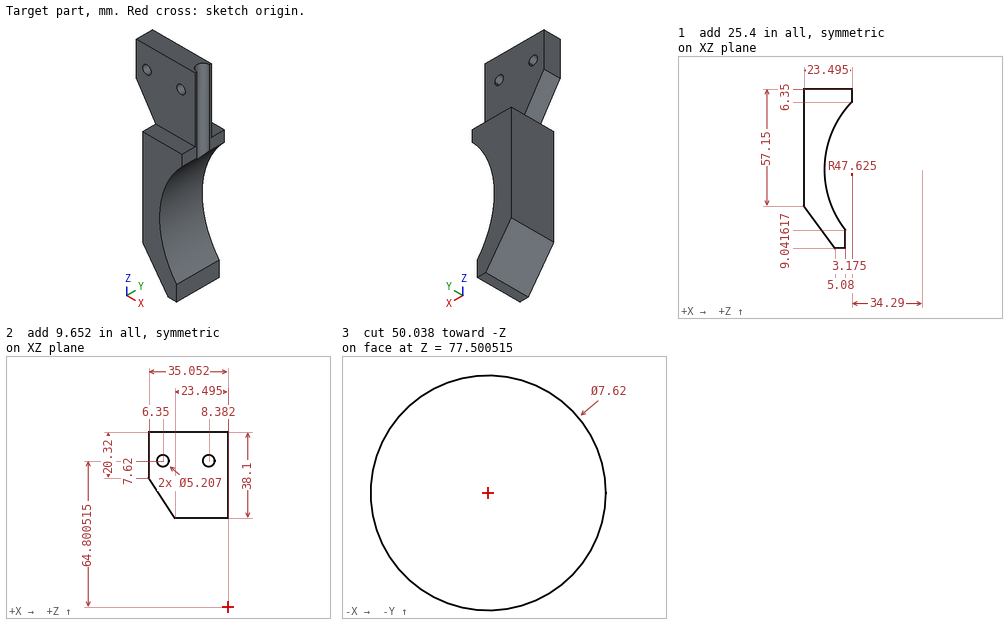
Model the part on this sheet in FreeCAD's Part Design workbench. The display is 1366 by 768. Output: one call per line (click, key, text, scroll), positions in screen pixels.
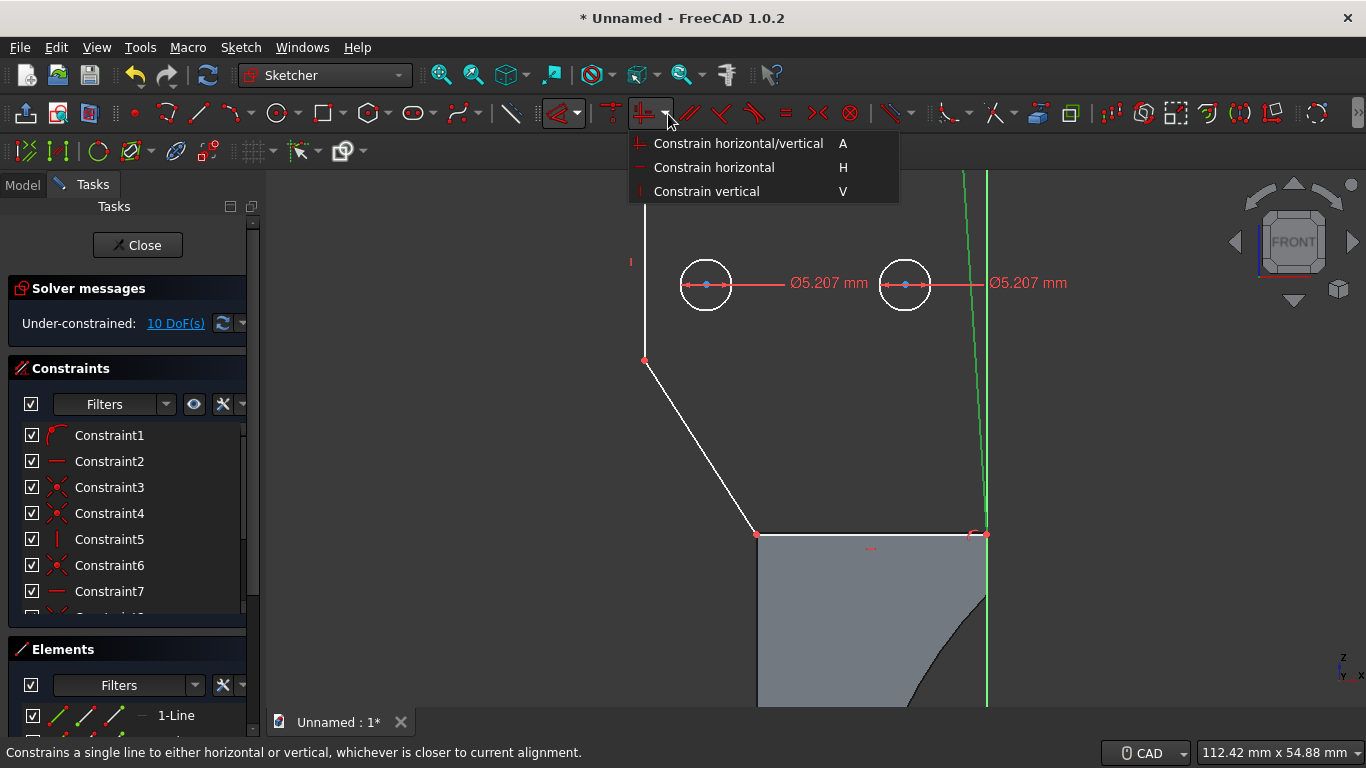
click(764, 191)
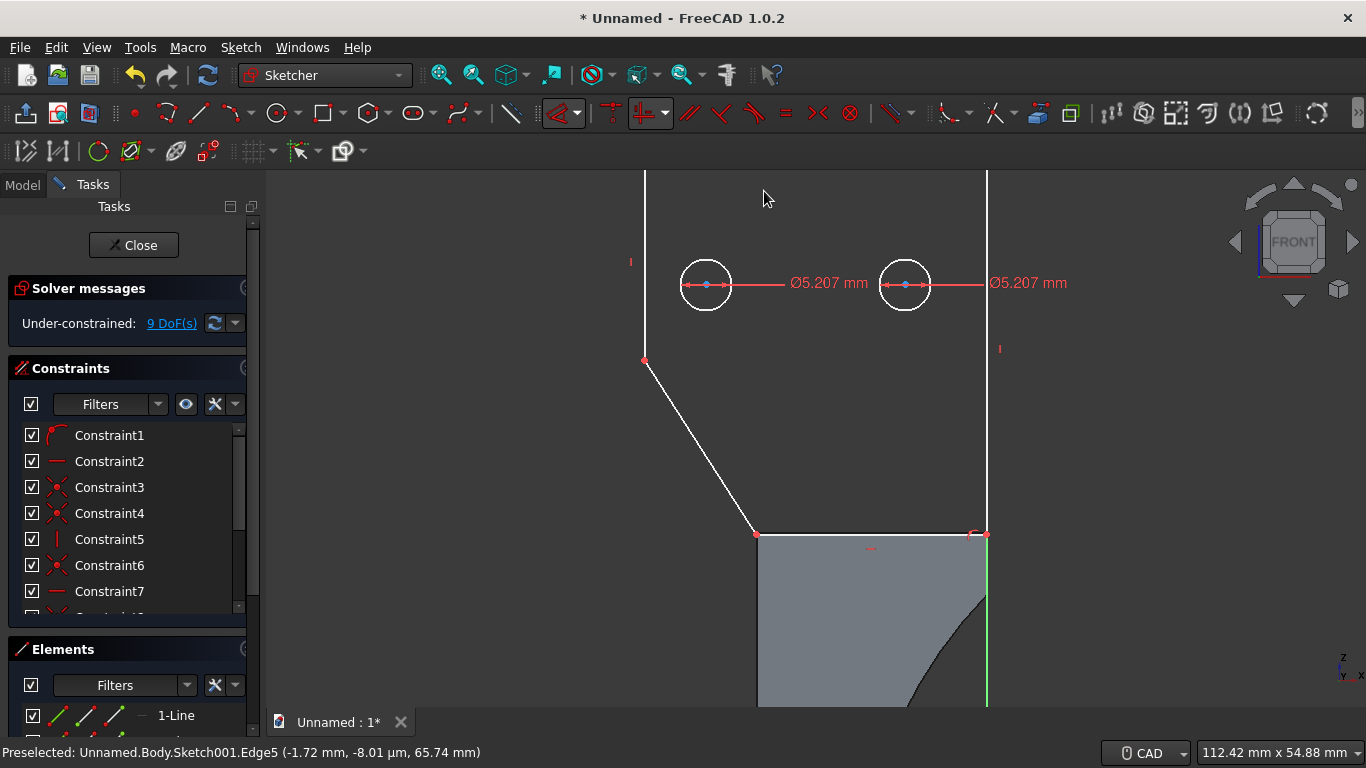
click(706, 285)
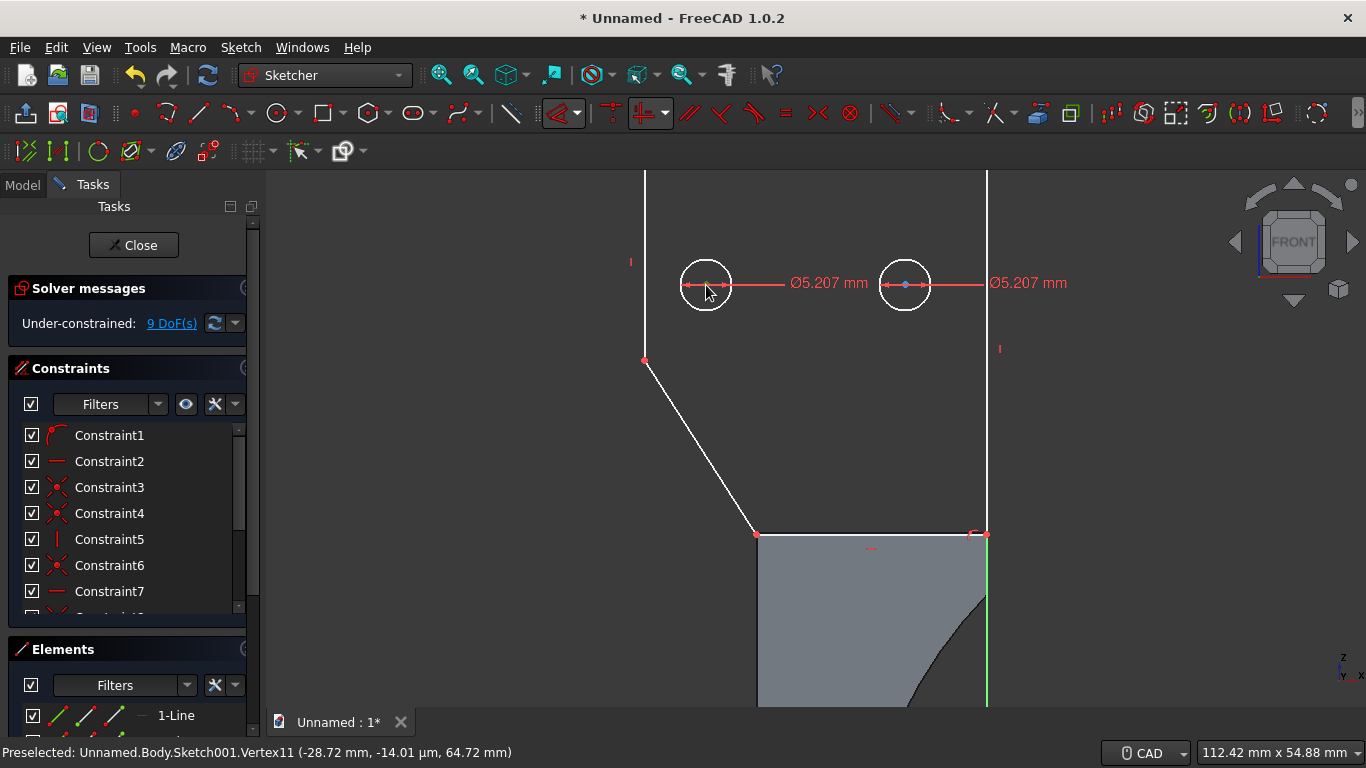
click(905, 285)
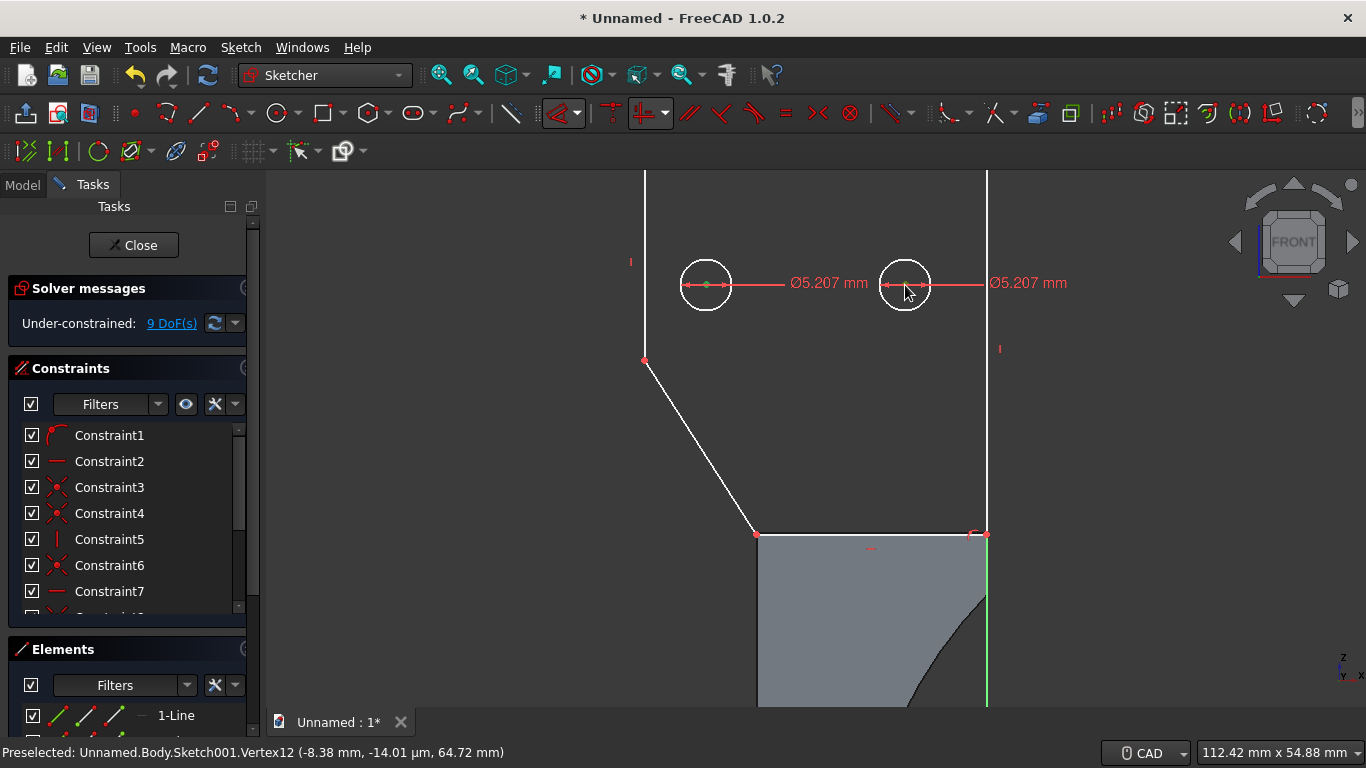
click(668, 114)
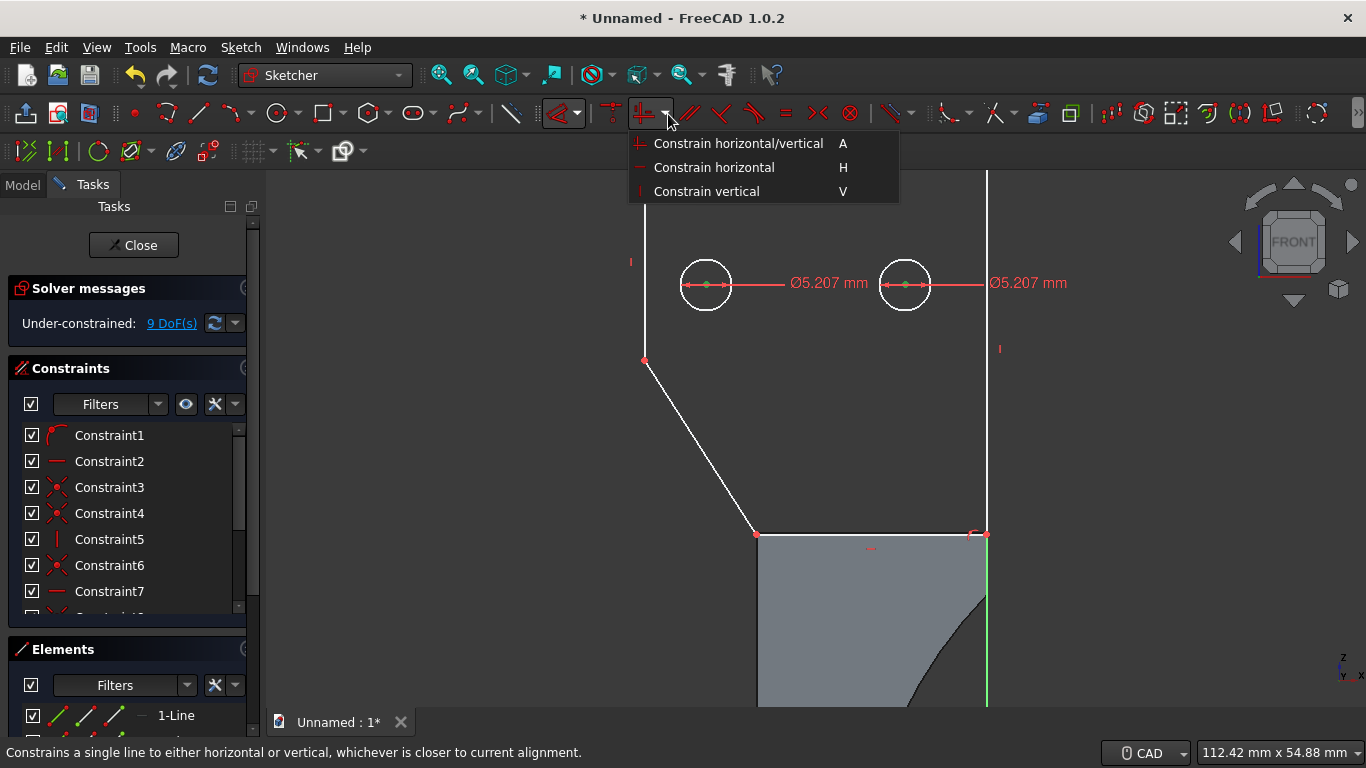
click(764, 167)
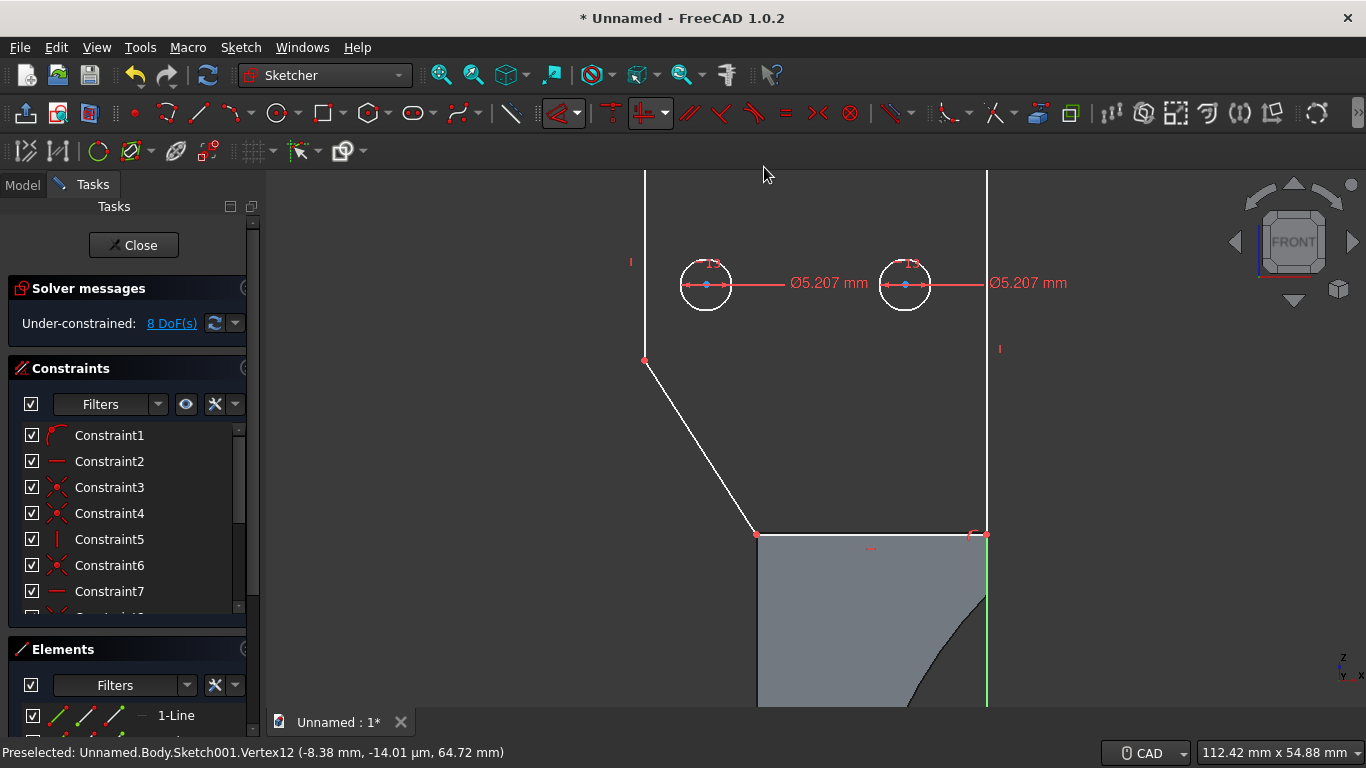
click(987, 274)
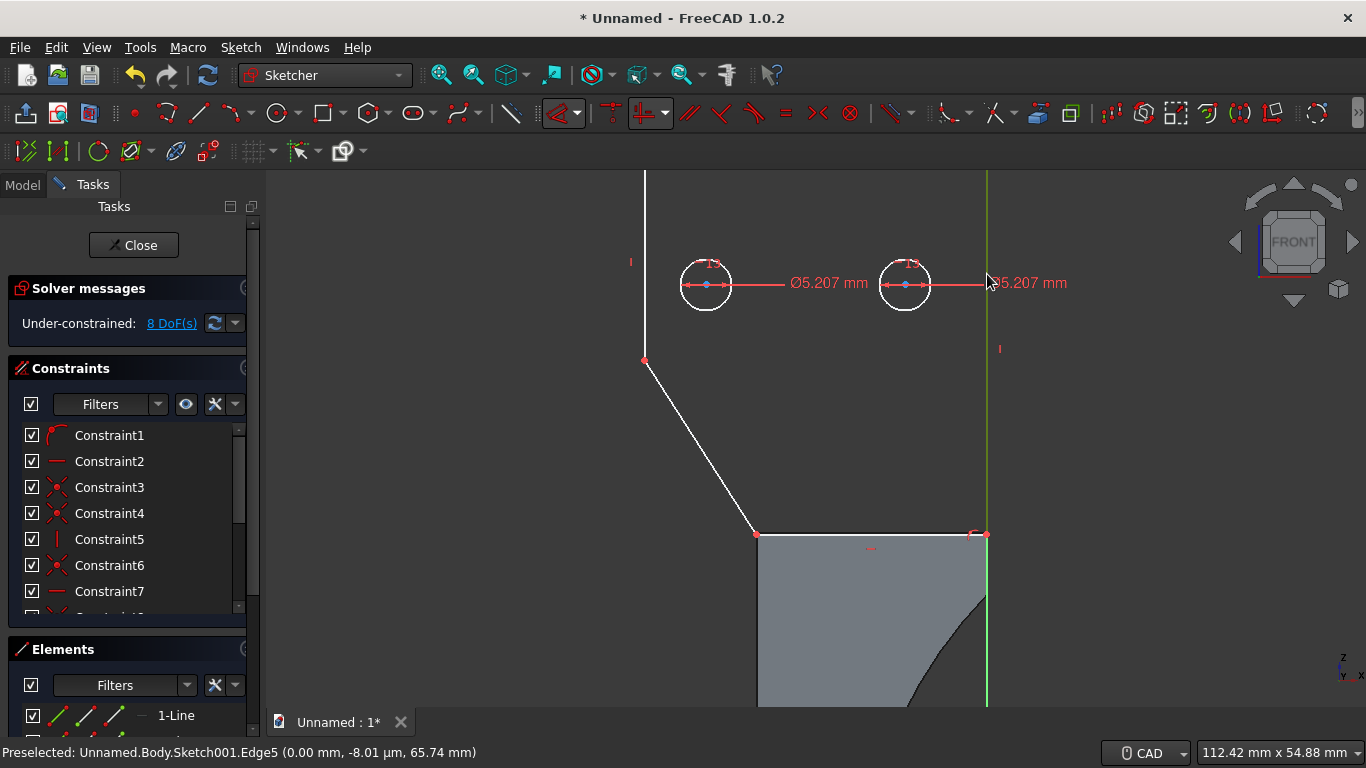
click(580, 114)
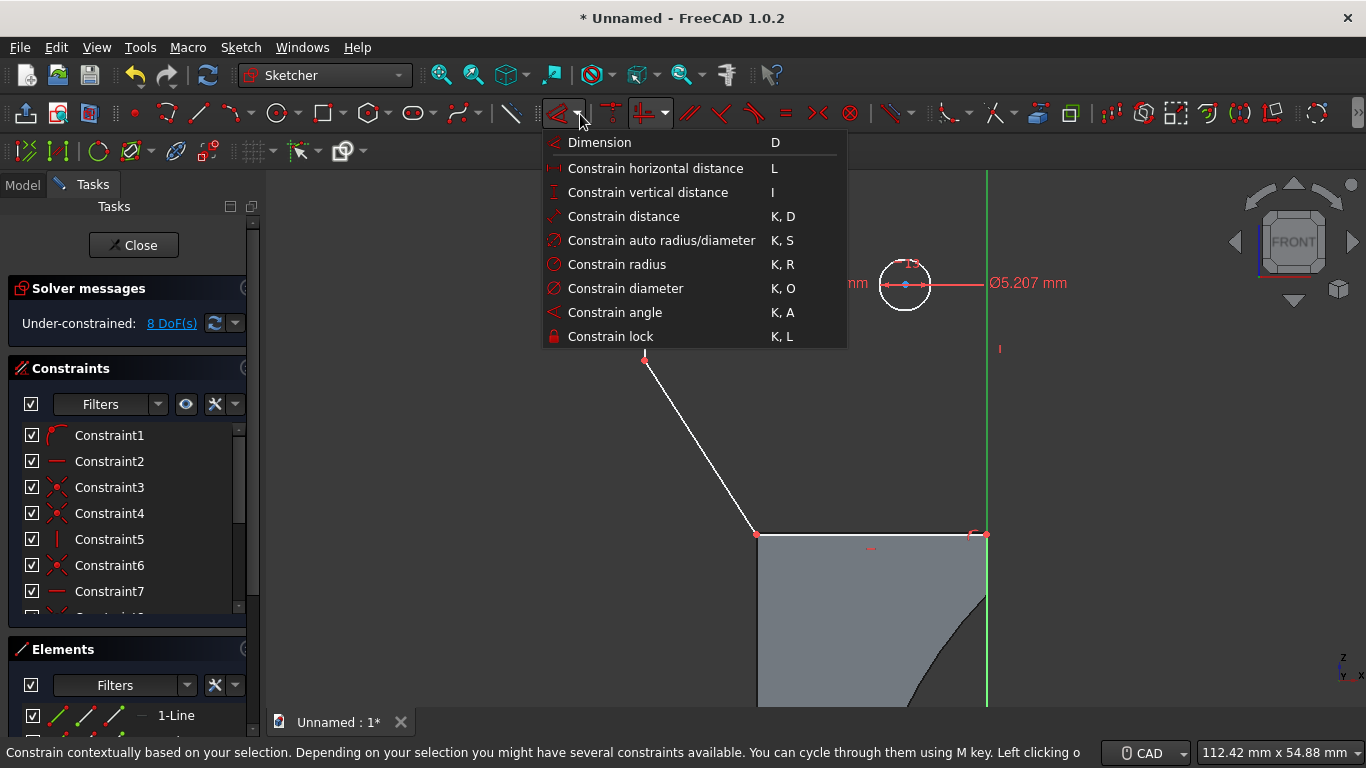
click(695, 192)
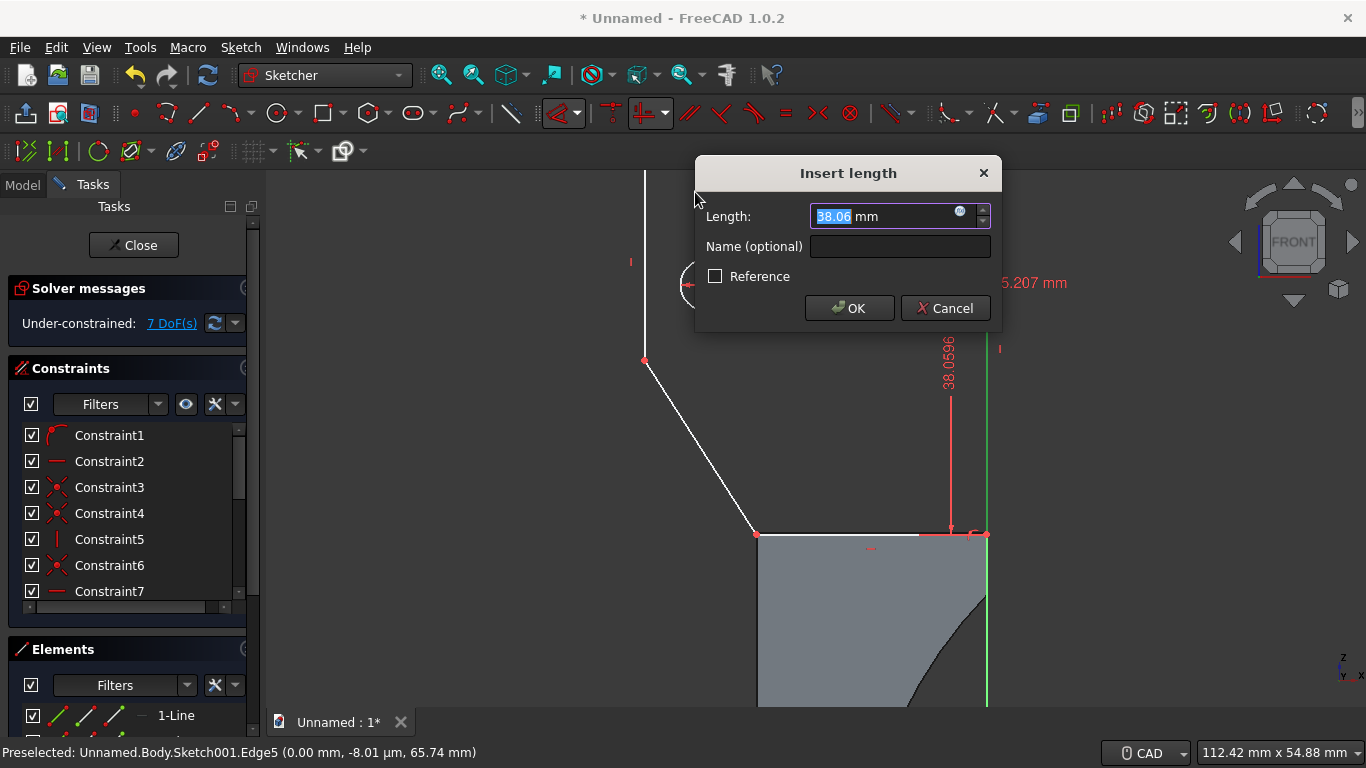
text(38.1)
key(Return)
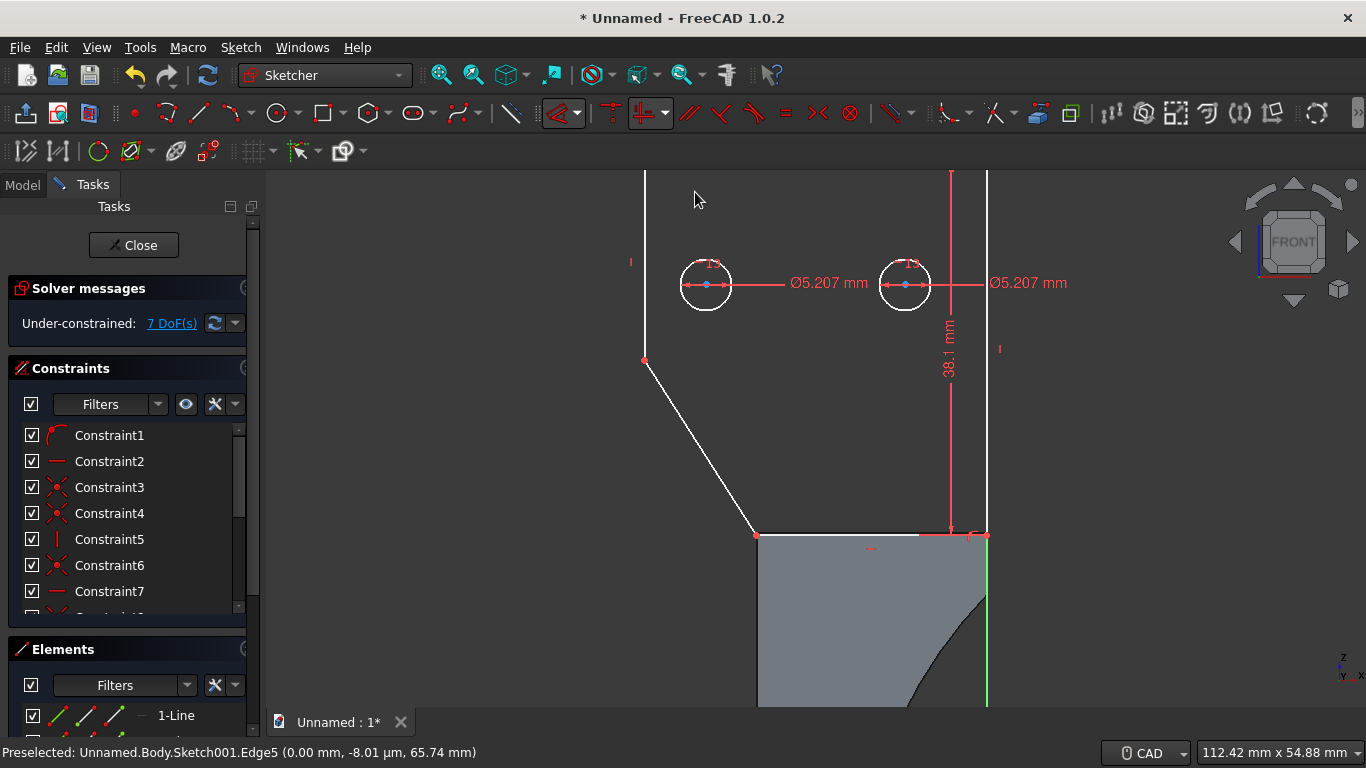
click(645, 301)